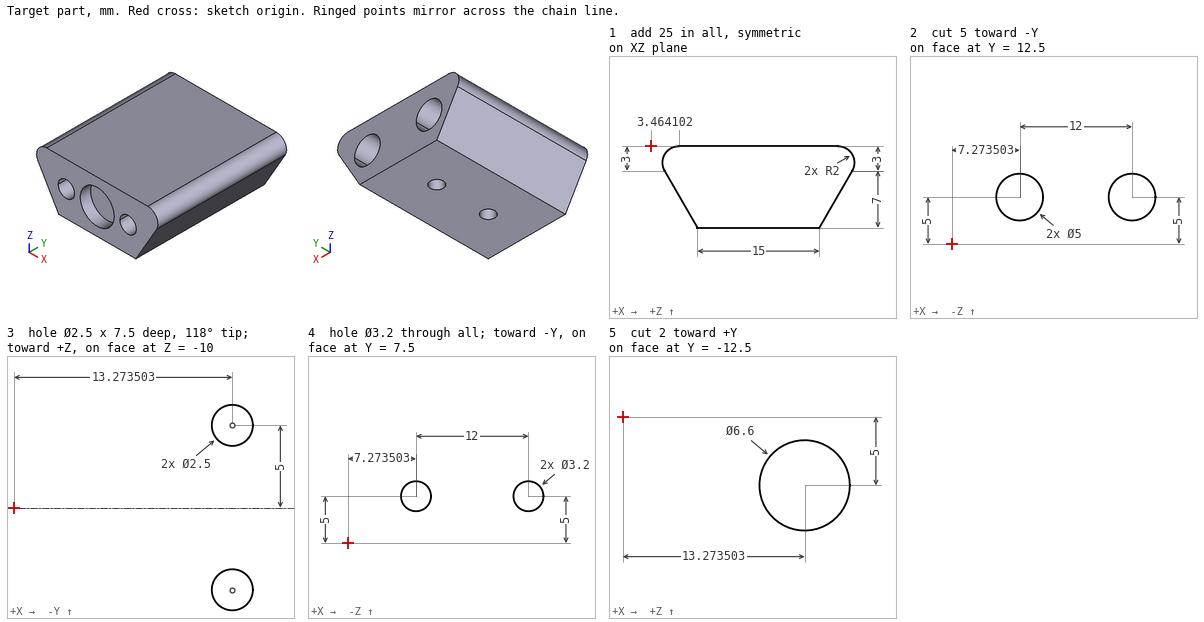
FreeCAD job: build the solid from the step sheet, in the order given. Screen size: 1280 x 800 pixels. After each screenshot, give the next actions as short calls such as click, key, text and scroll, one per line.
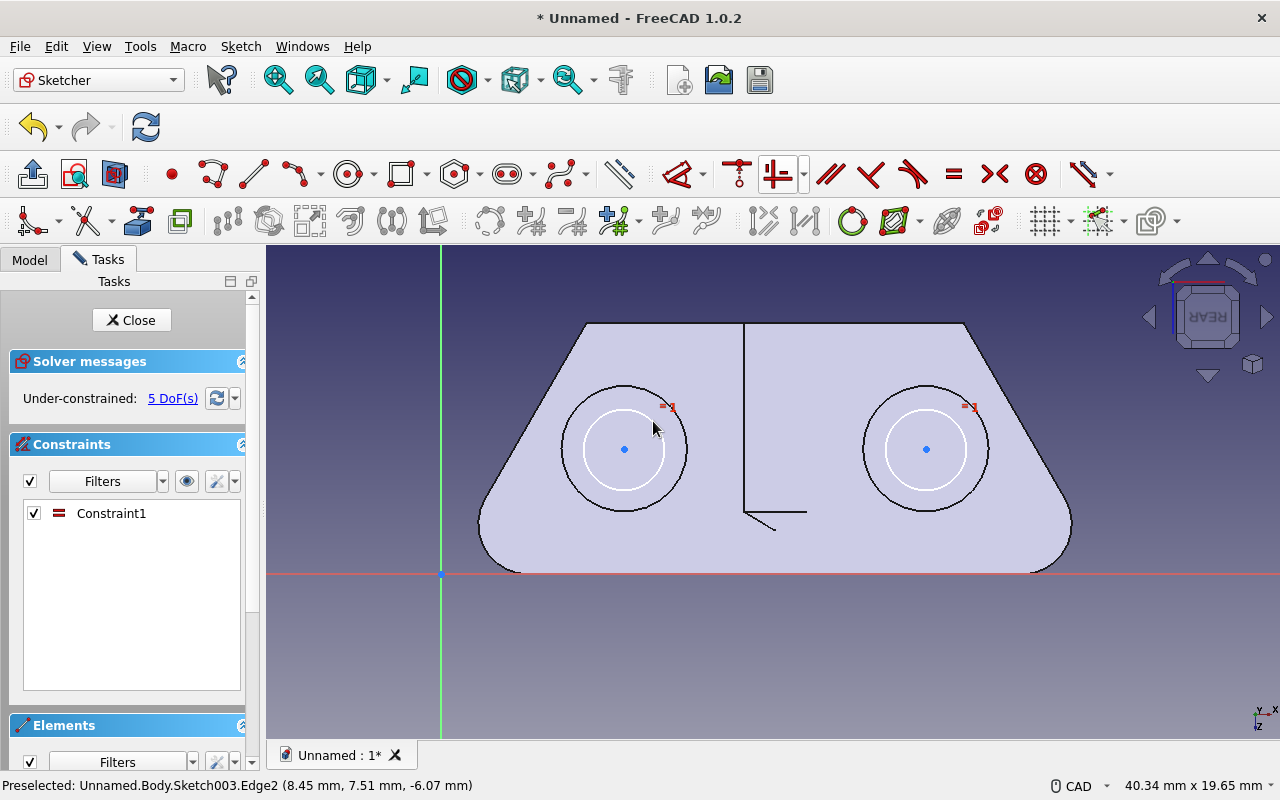
click(676, 174)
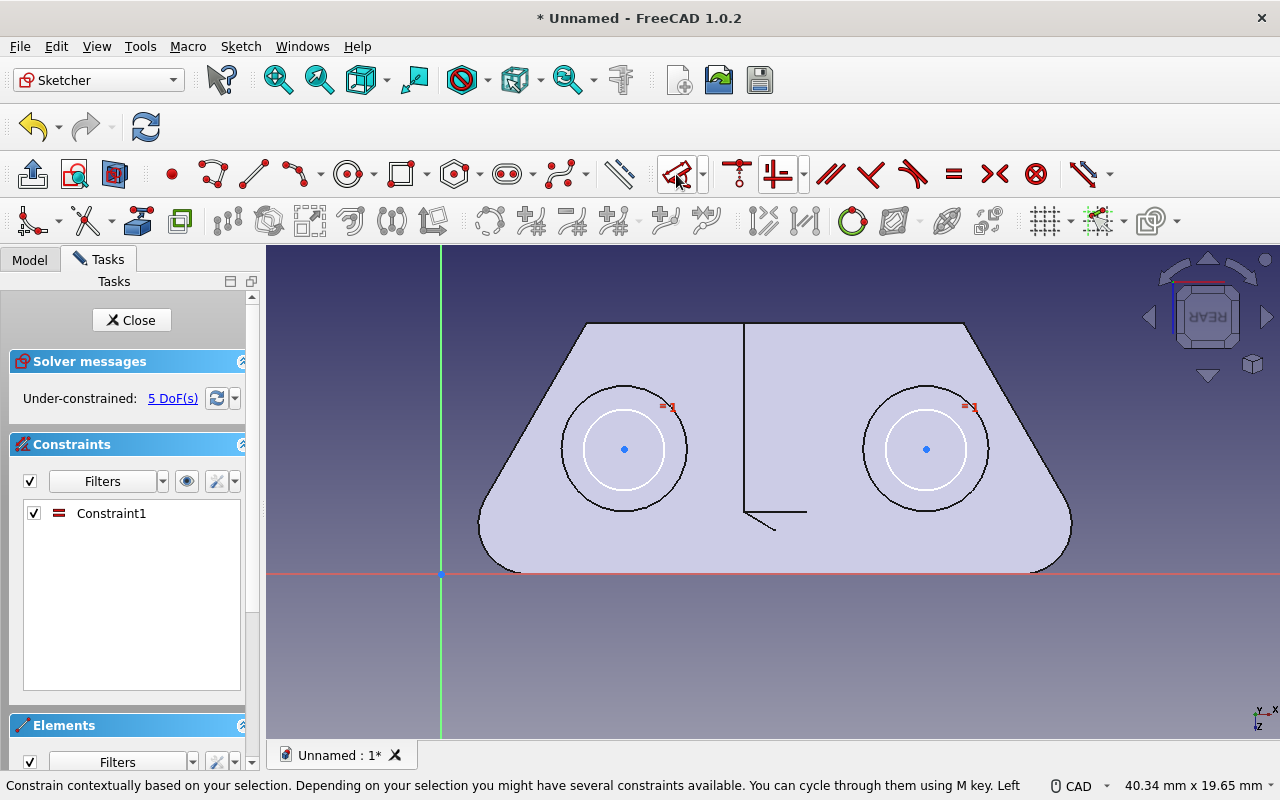
click(954, 421)
click(976, 398)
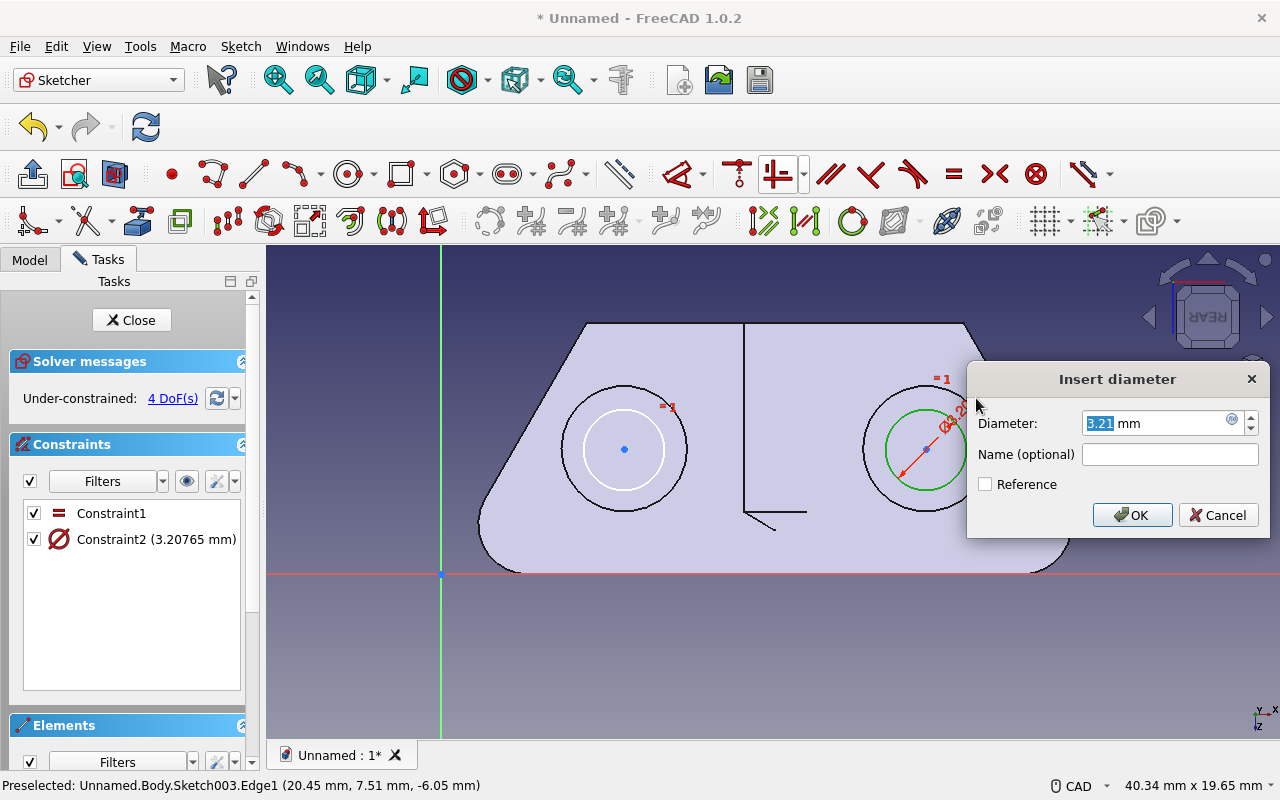
text(3.2)
key(Return)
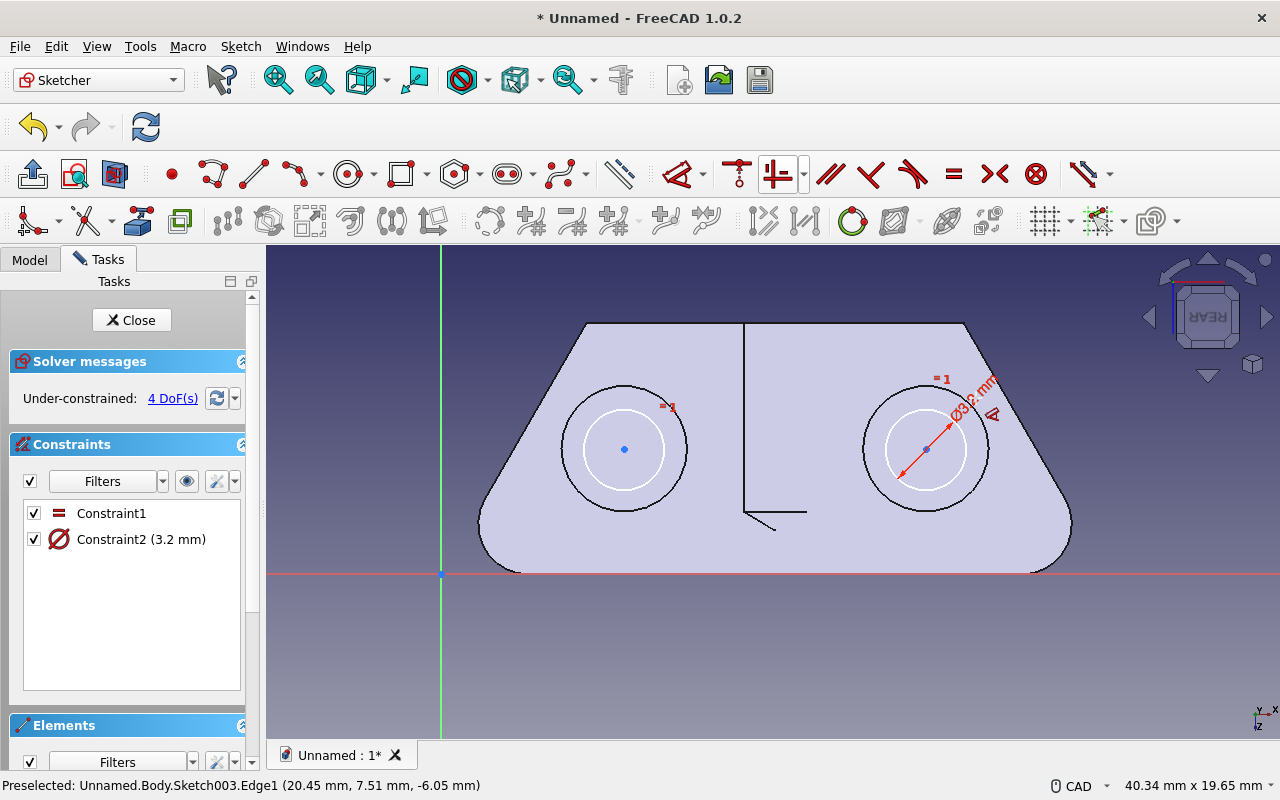
click(926, 450)
click(407, 512)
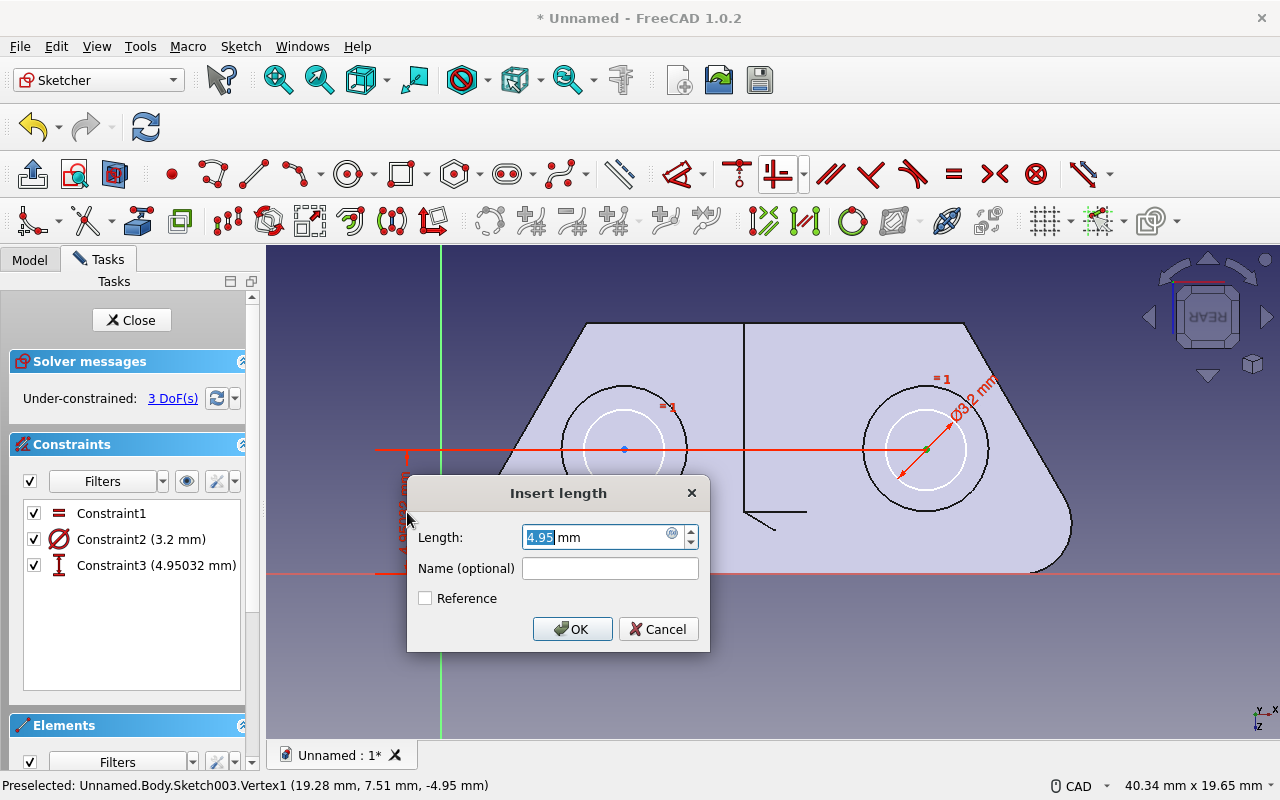
text(5)
key(Return)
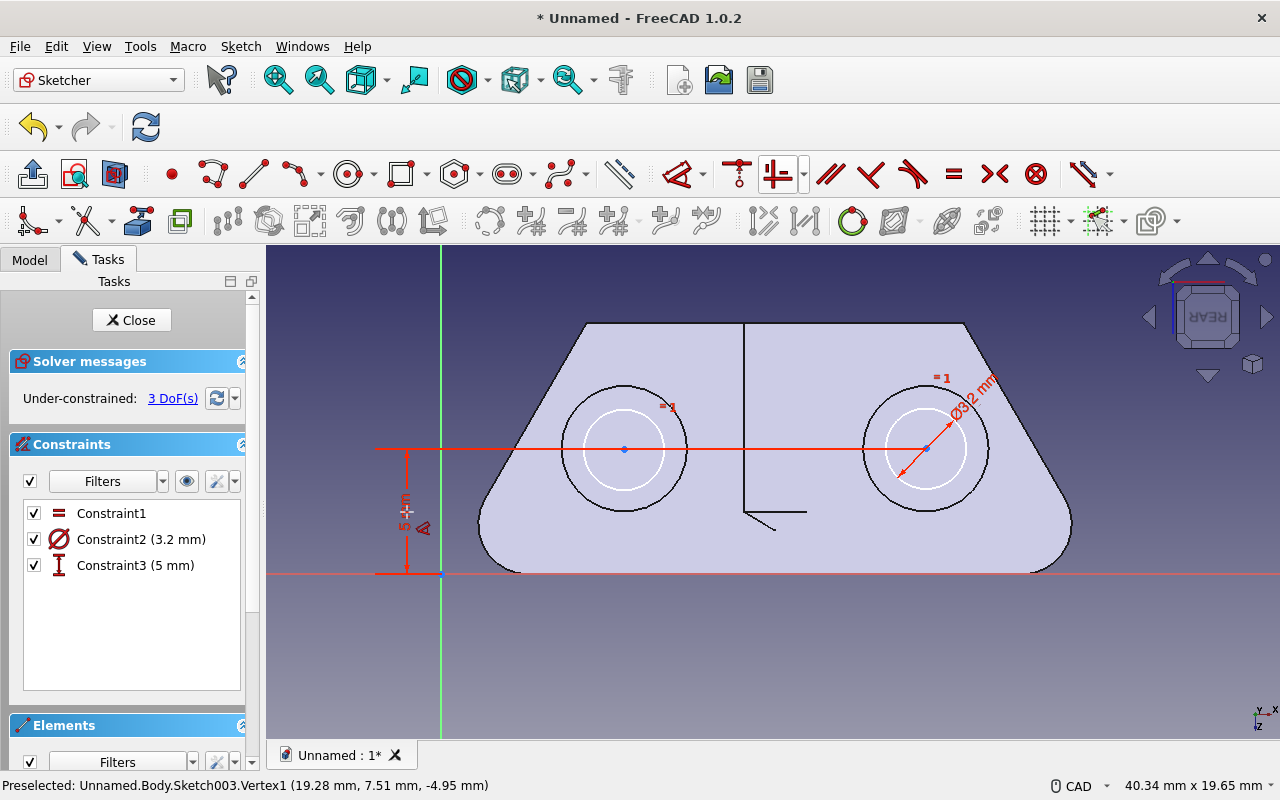
click(624, 450)
click(407, 484)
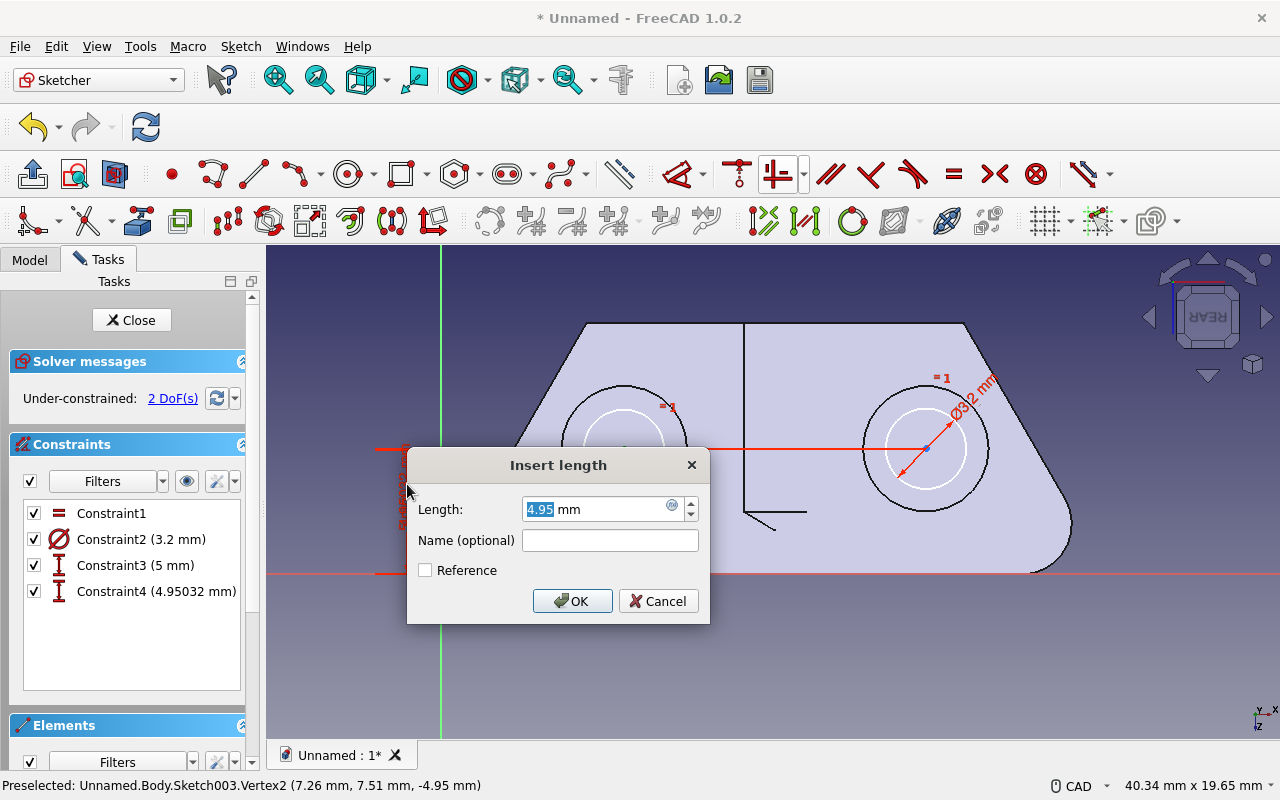
text(5)
key(Return)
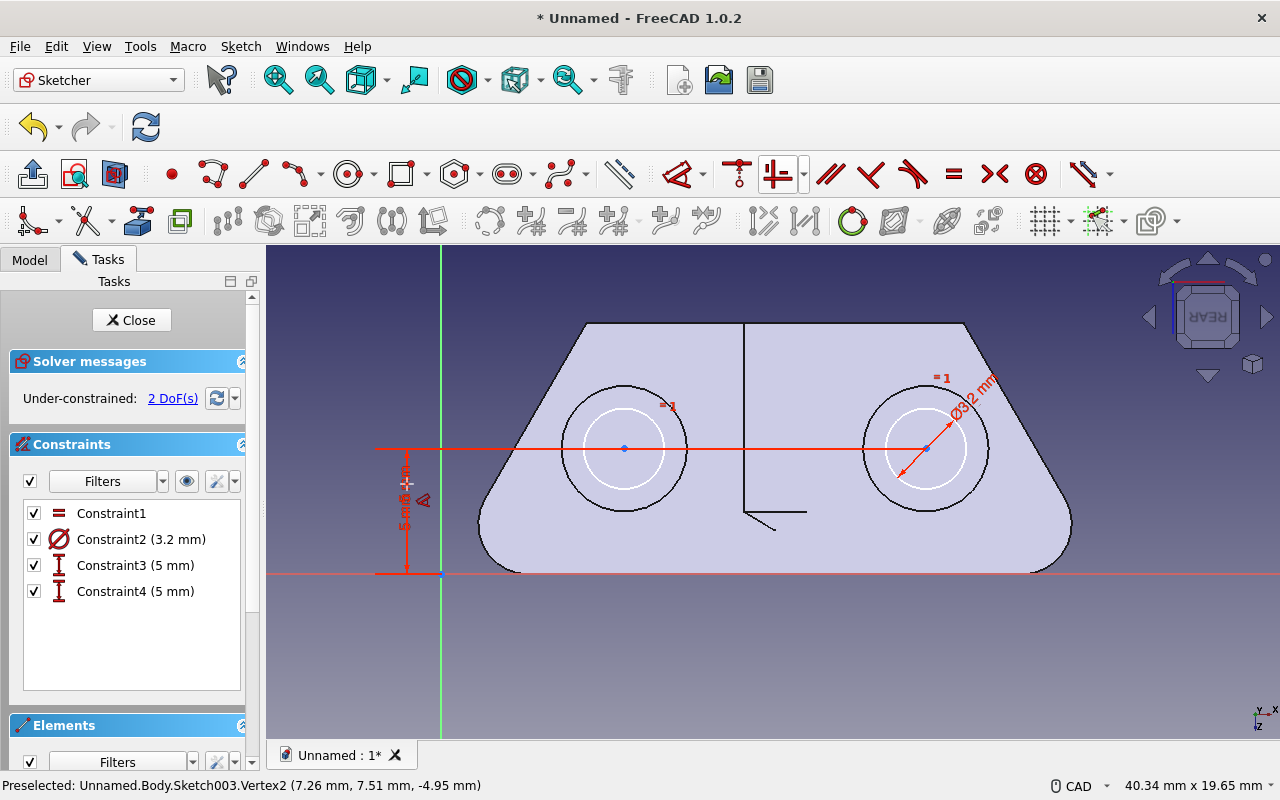
click(926, 449)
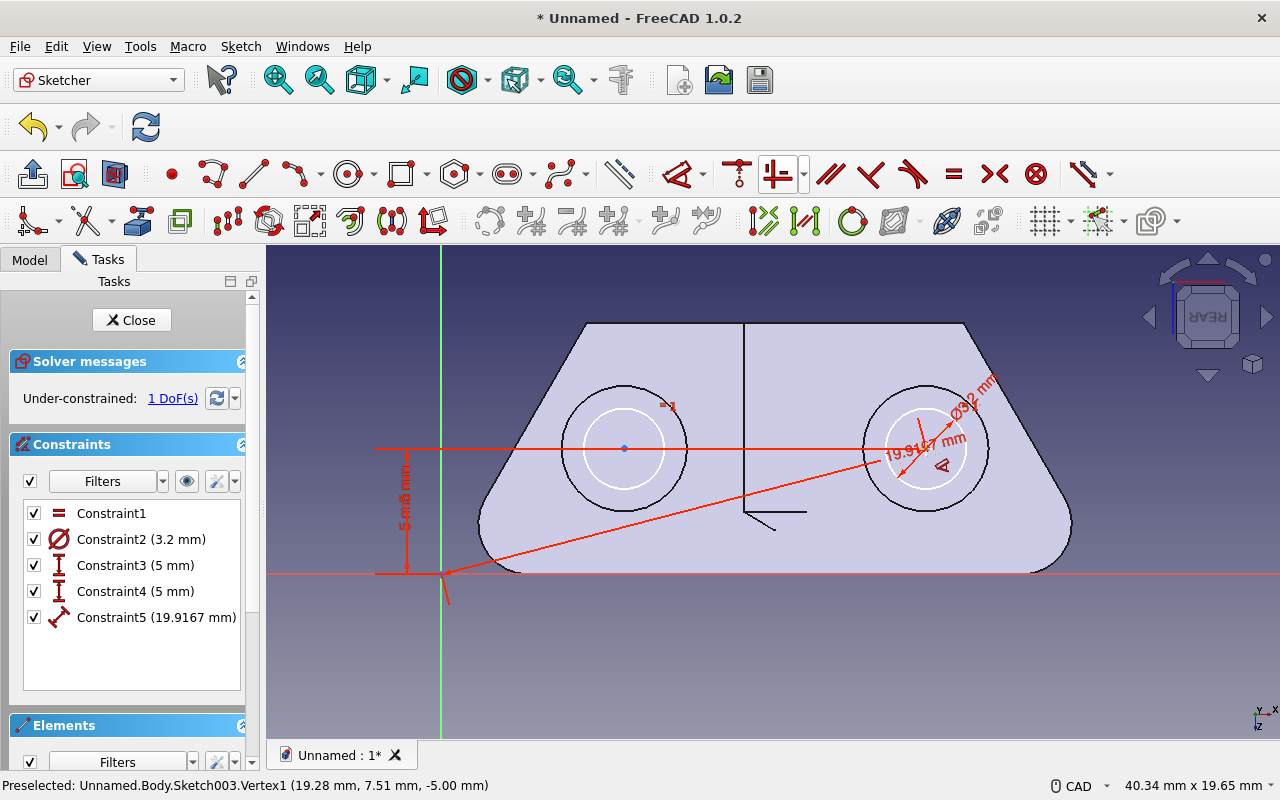
click(624, 449)
click(775, 415)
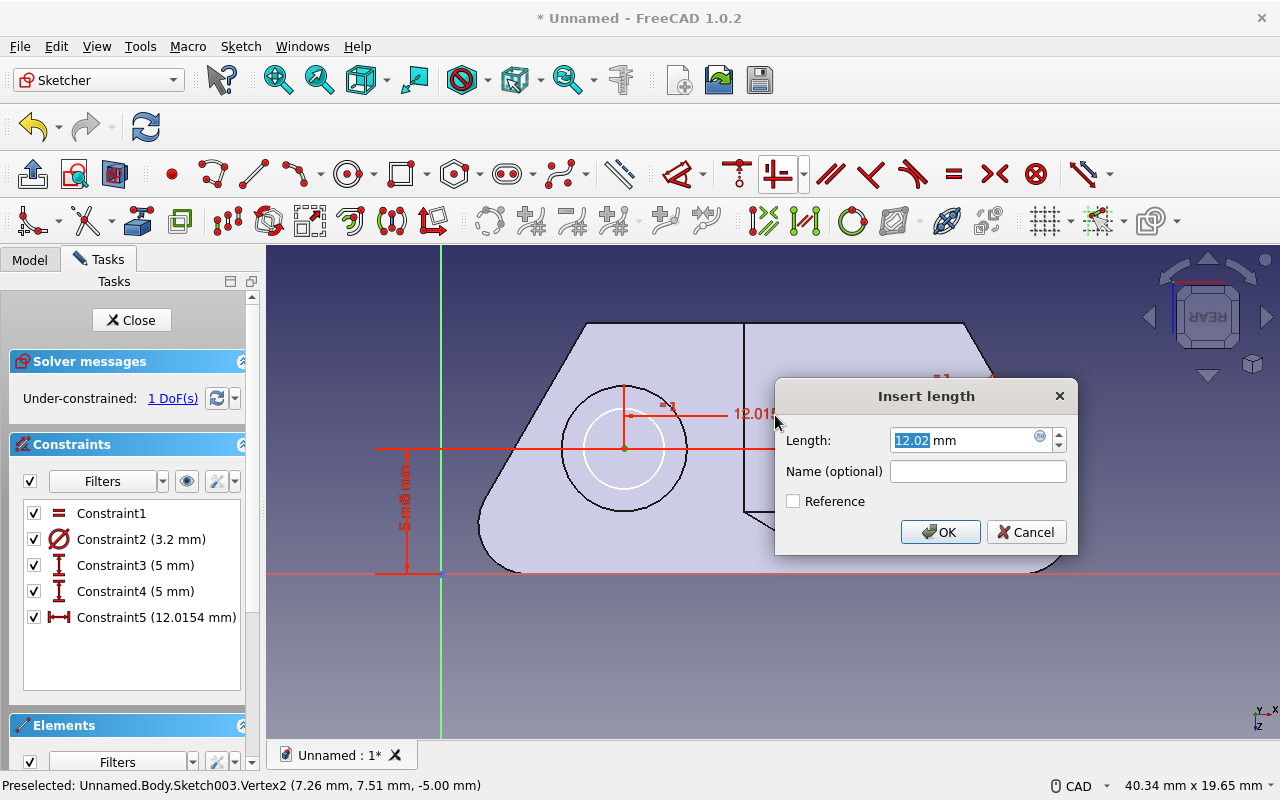
text(12)
key(Return)